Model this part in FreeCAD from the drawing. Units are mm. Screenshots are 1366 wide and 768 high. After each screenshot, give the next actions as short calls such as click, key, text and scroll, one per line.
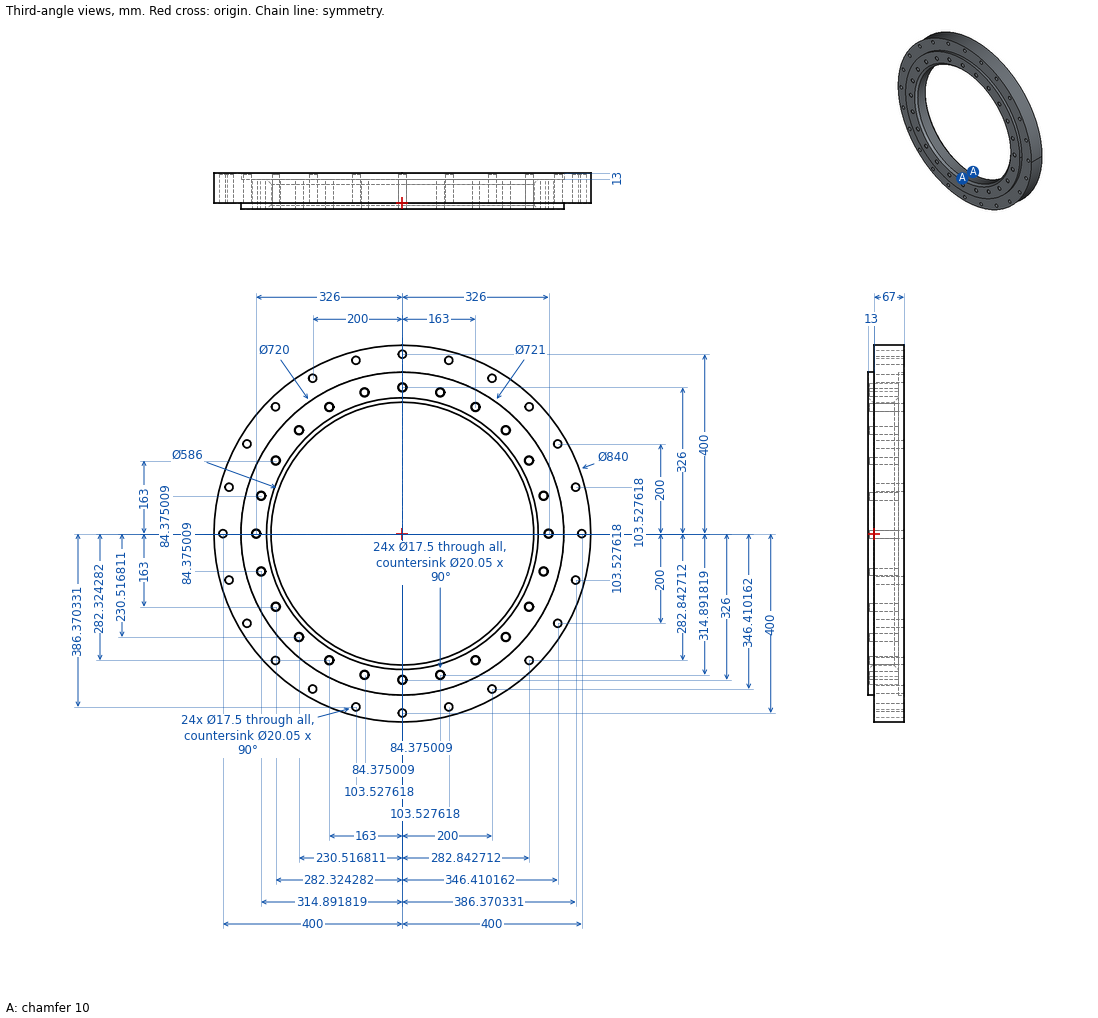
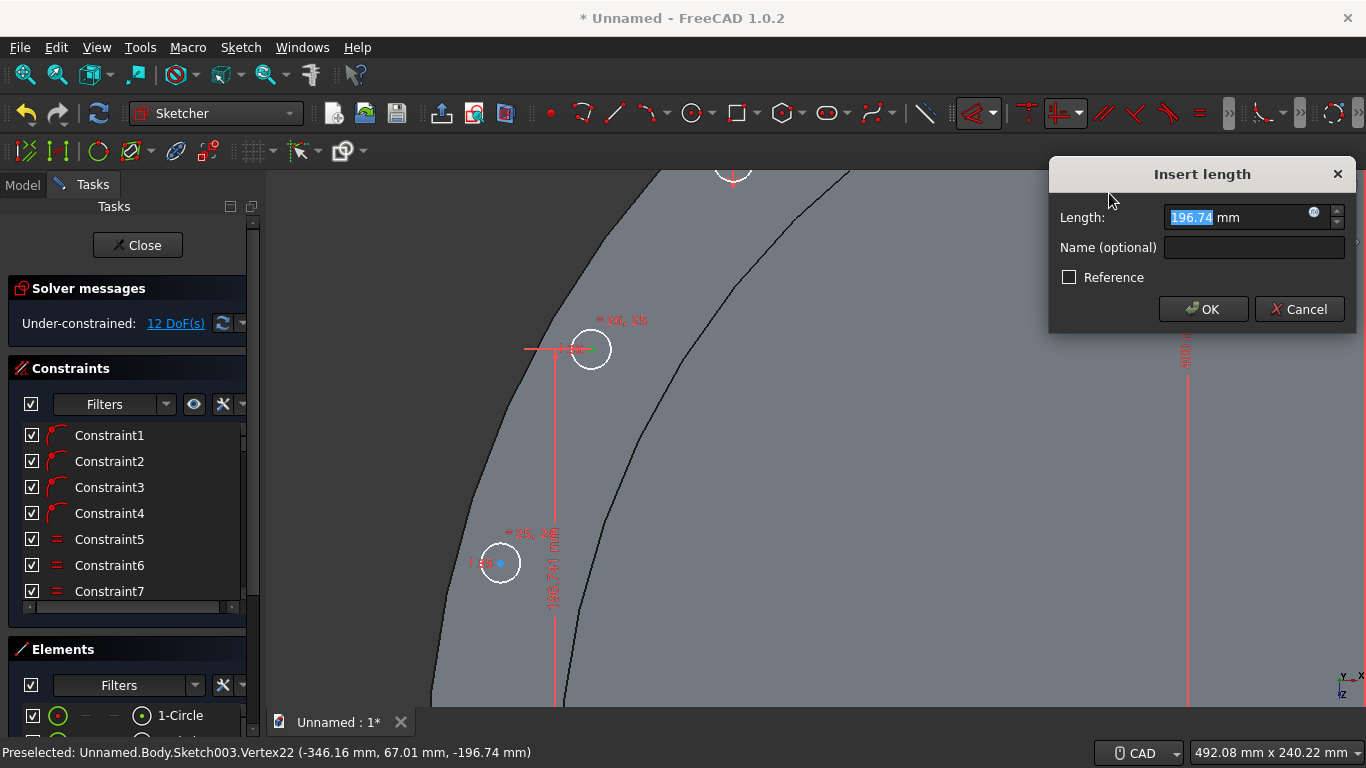
text(200)
key(Return)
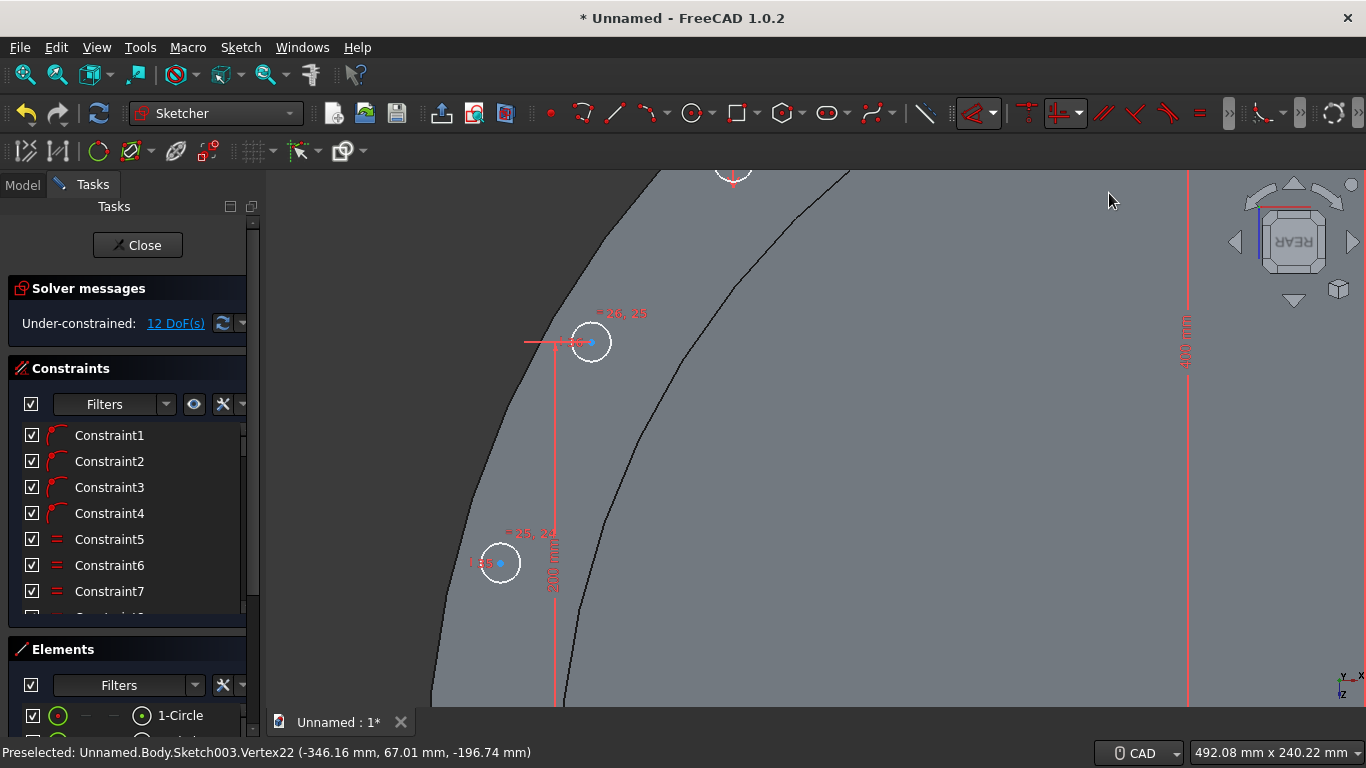
scroll(591, 350, down, 8)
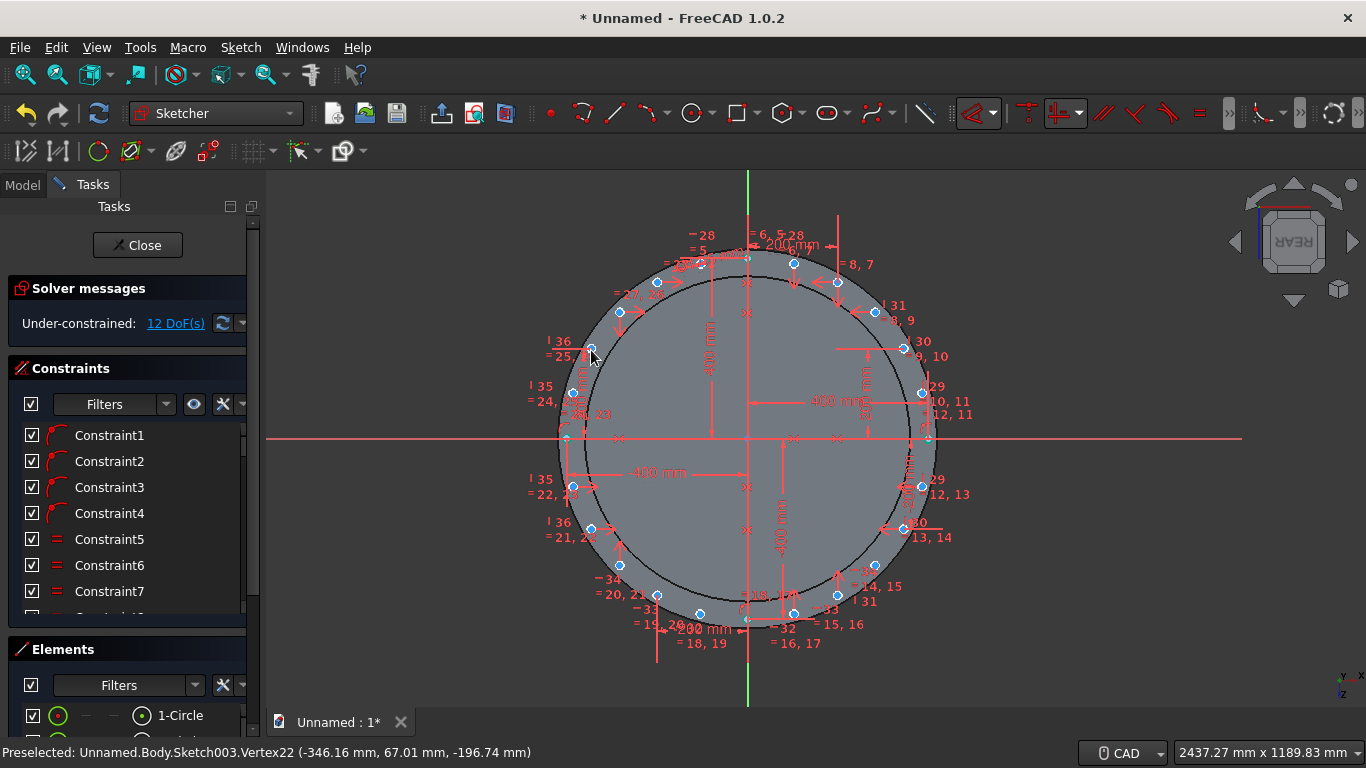
click(701, 264)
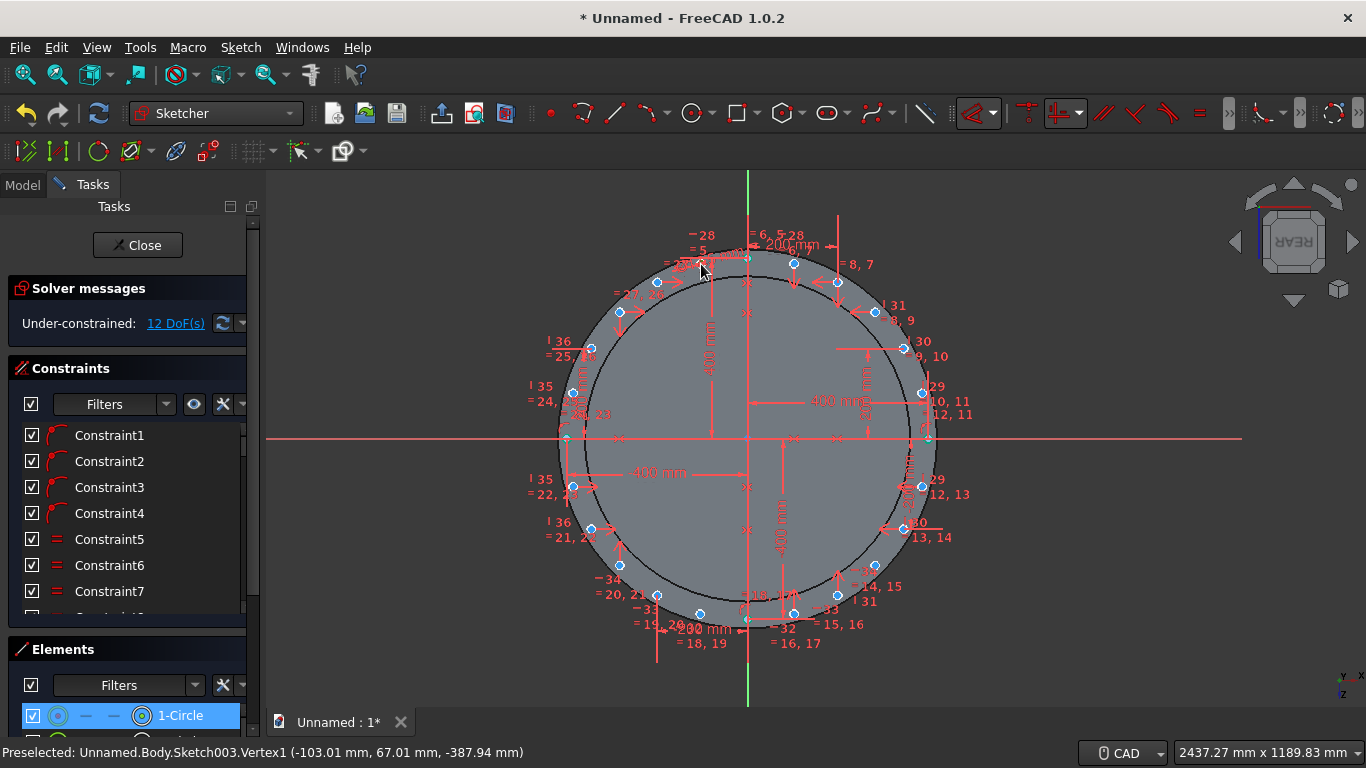
key(l)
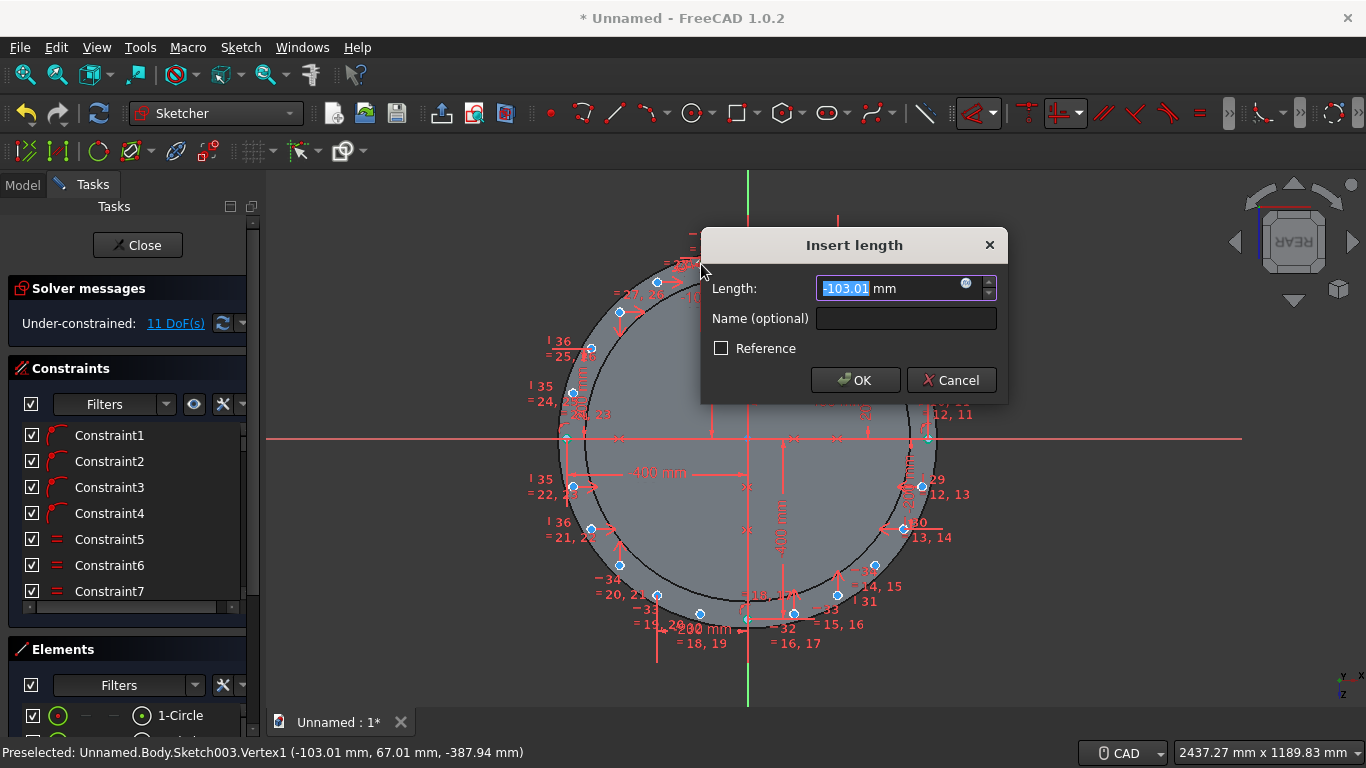
text(-103.527618)
key(Return)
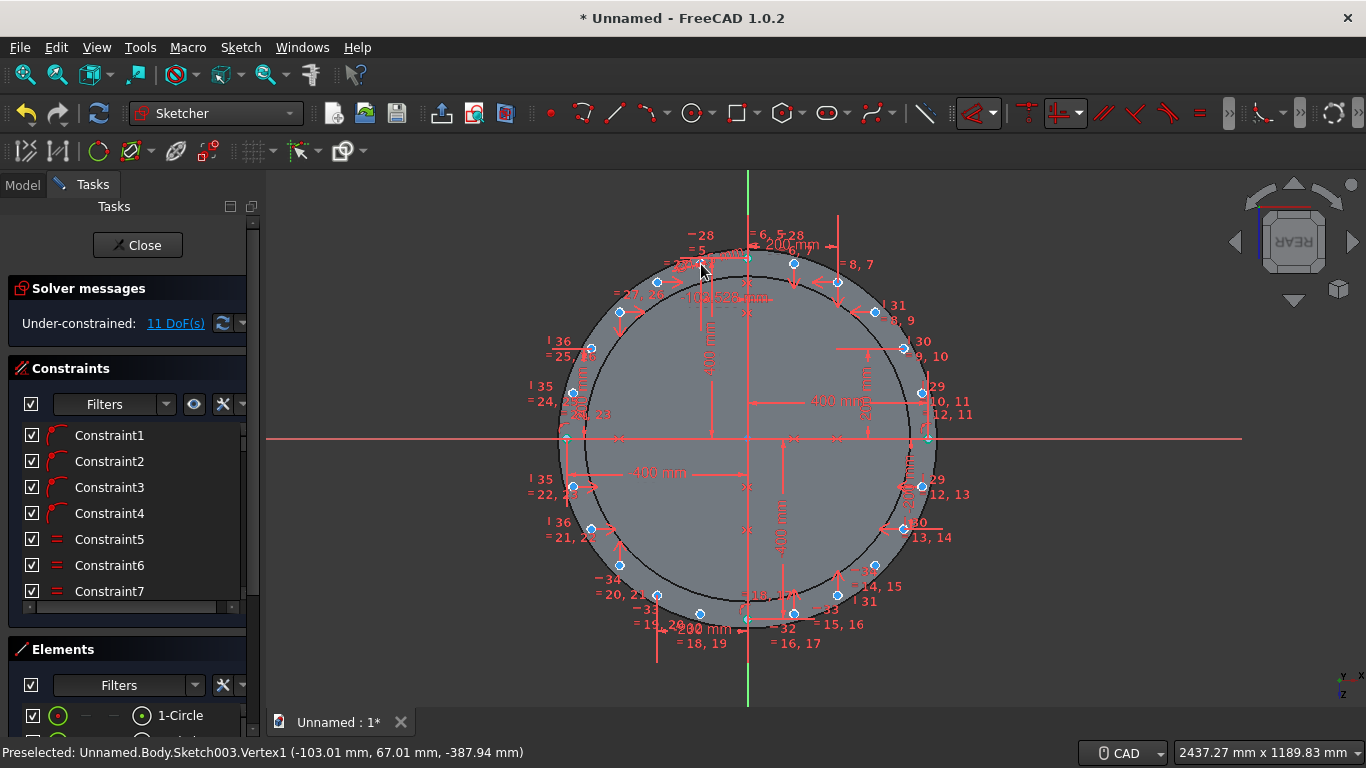
click(701, 264)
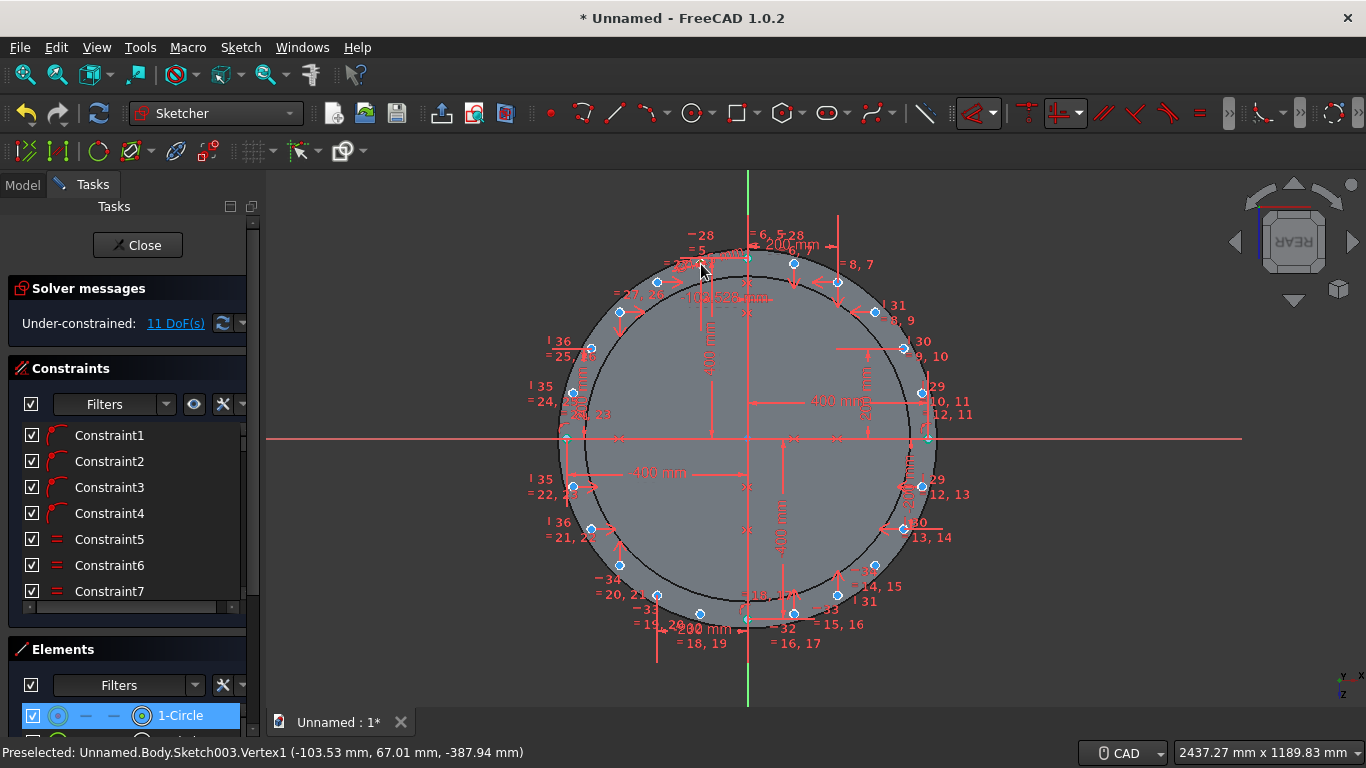
key(i)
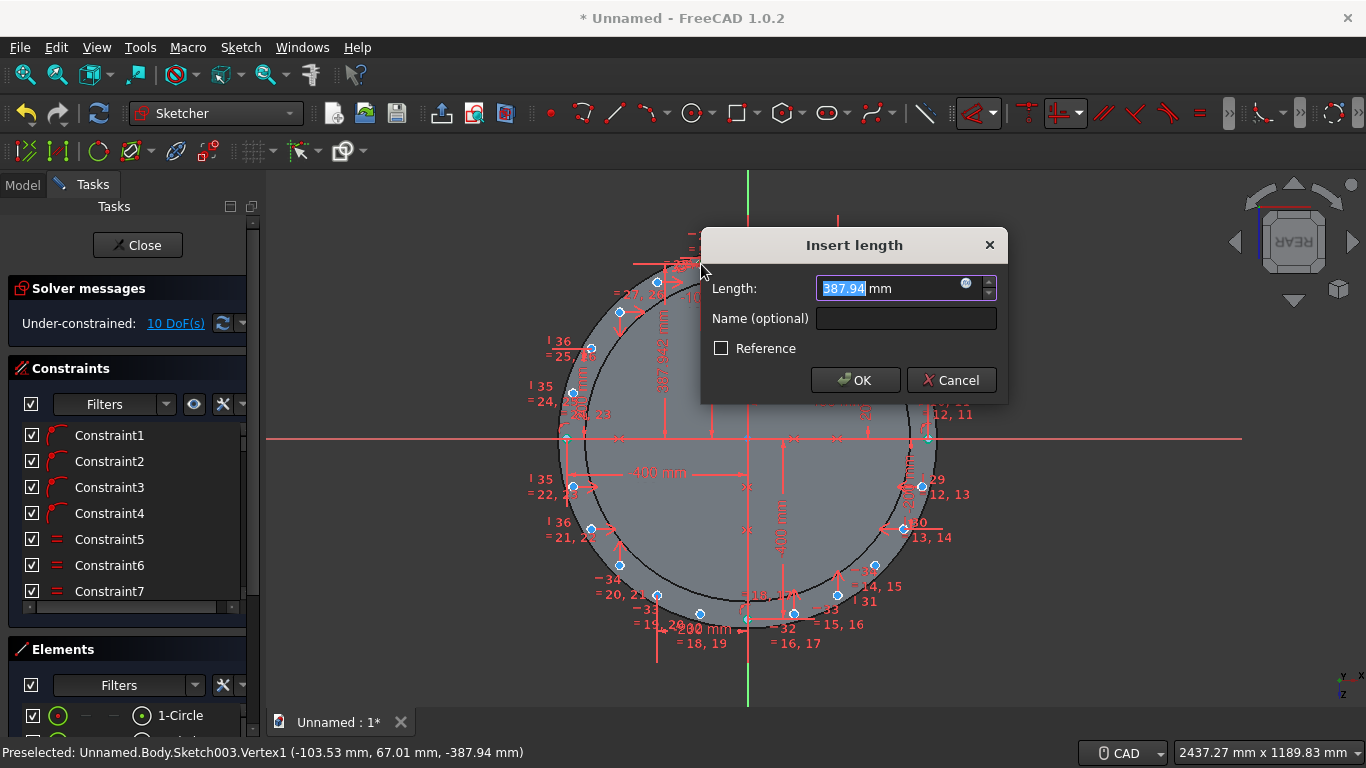
text(386.370331)
key(Return)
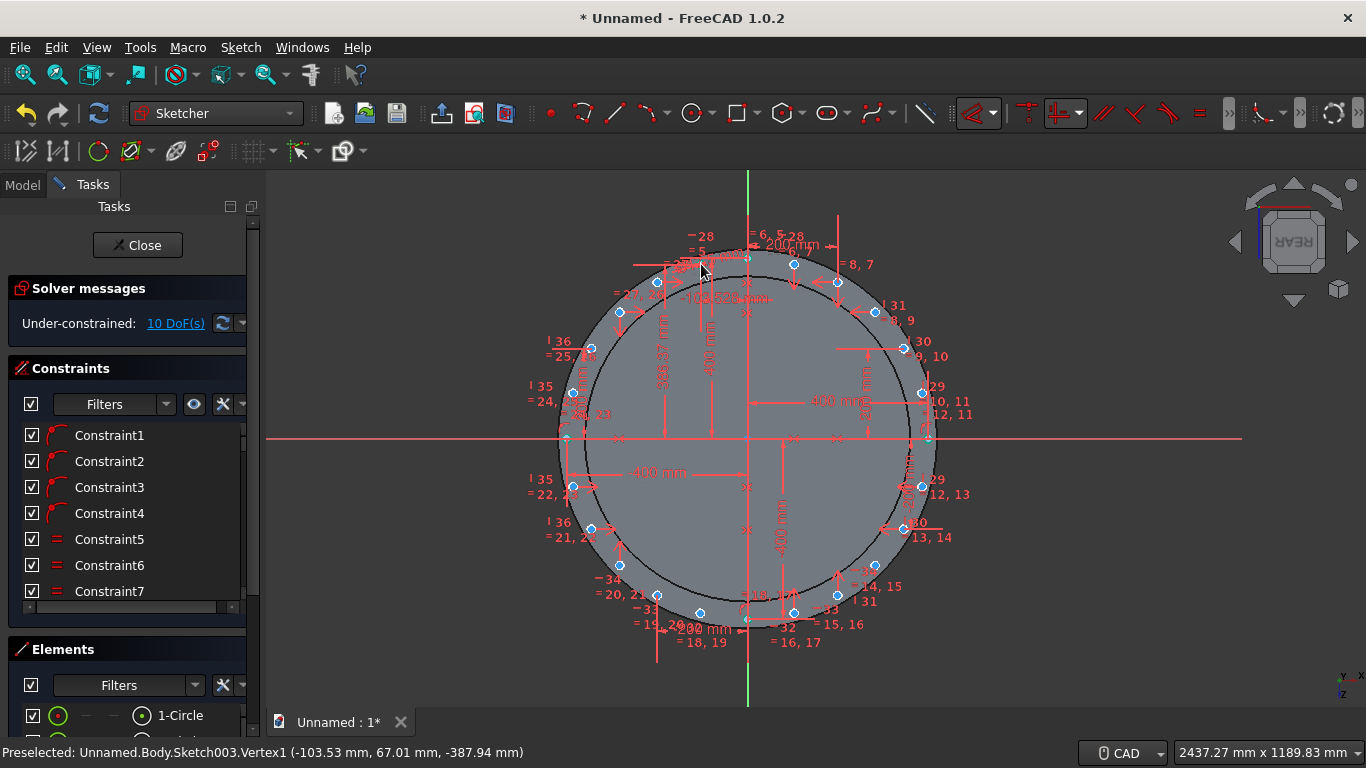
click(794, 265)